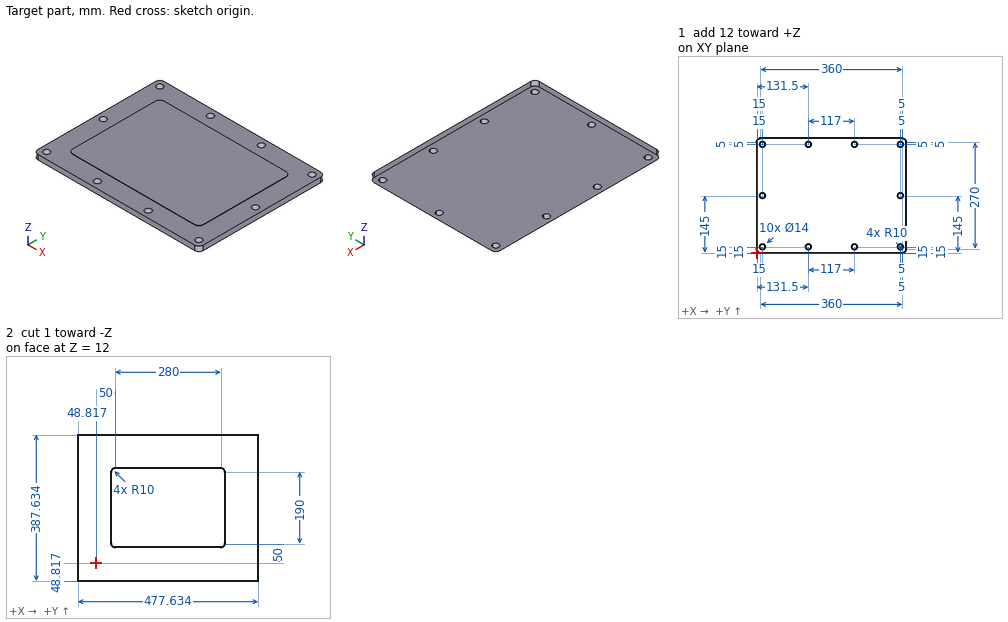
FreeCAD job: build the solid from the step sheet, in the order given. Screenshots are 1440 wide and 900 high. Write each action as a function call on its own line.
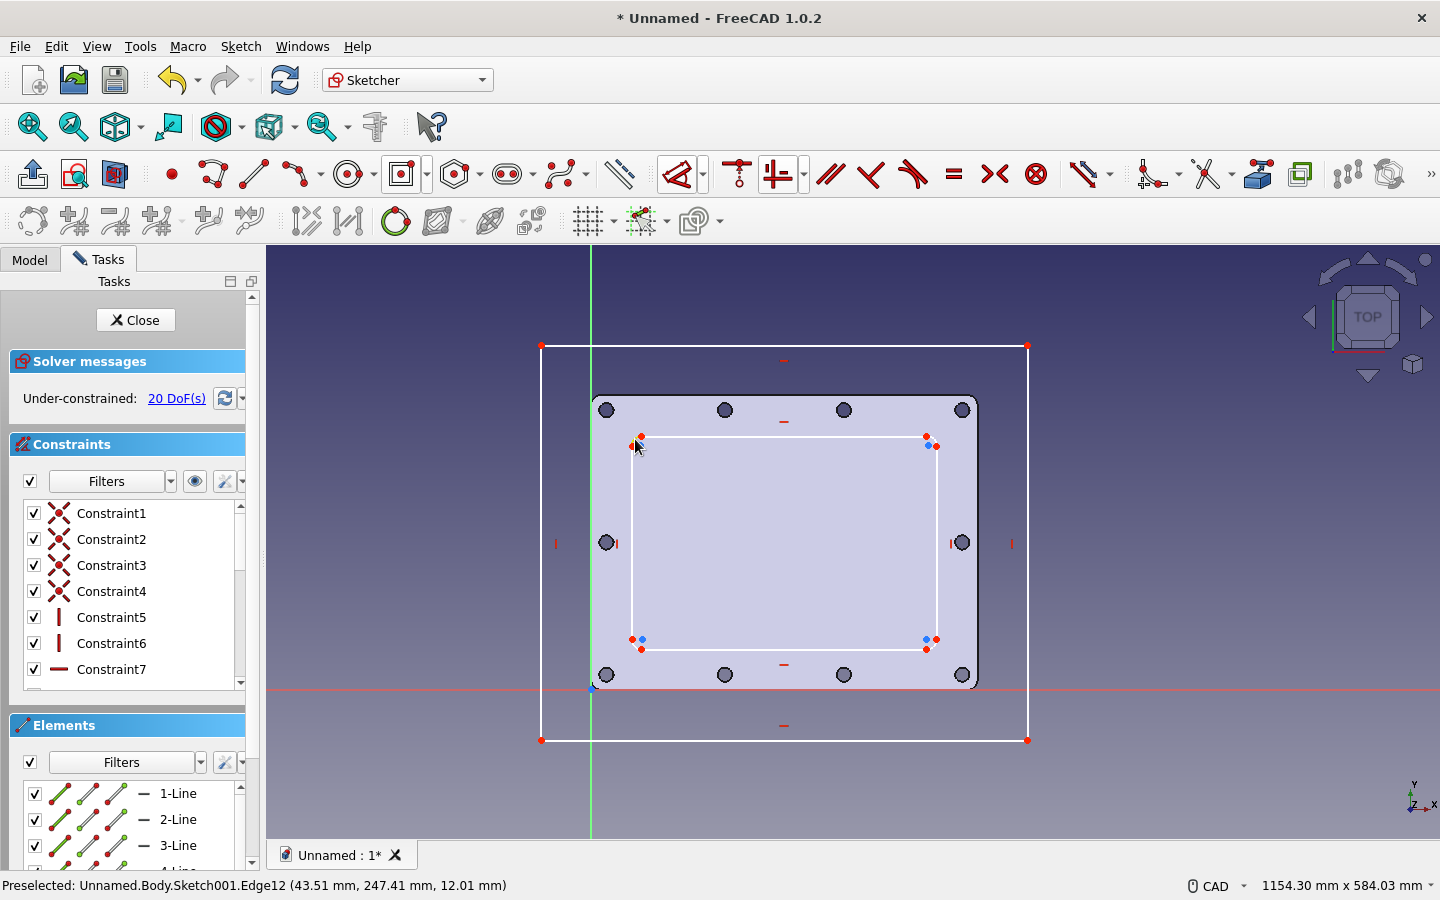
click(727, 437)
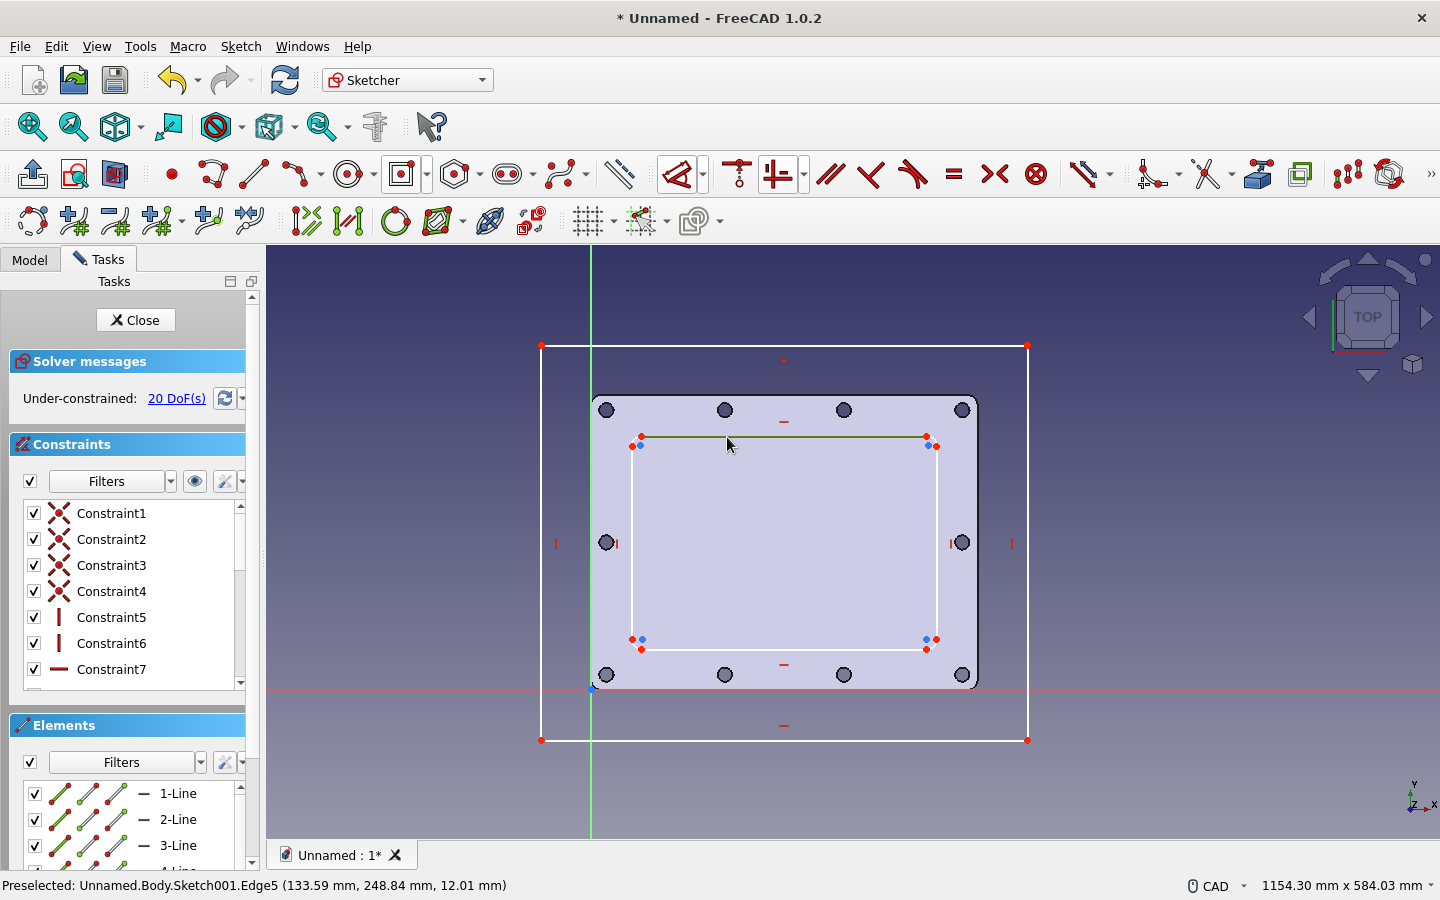
scroll(934, 439, up, 3)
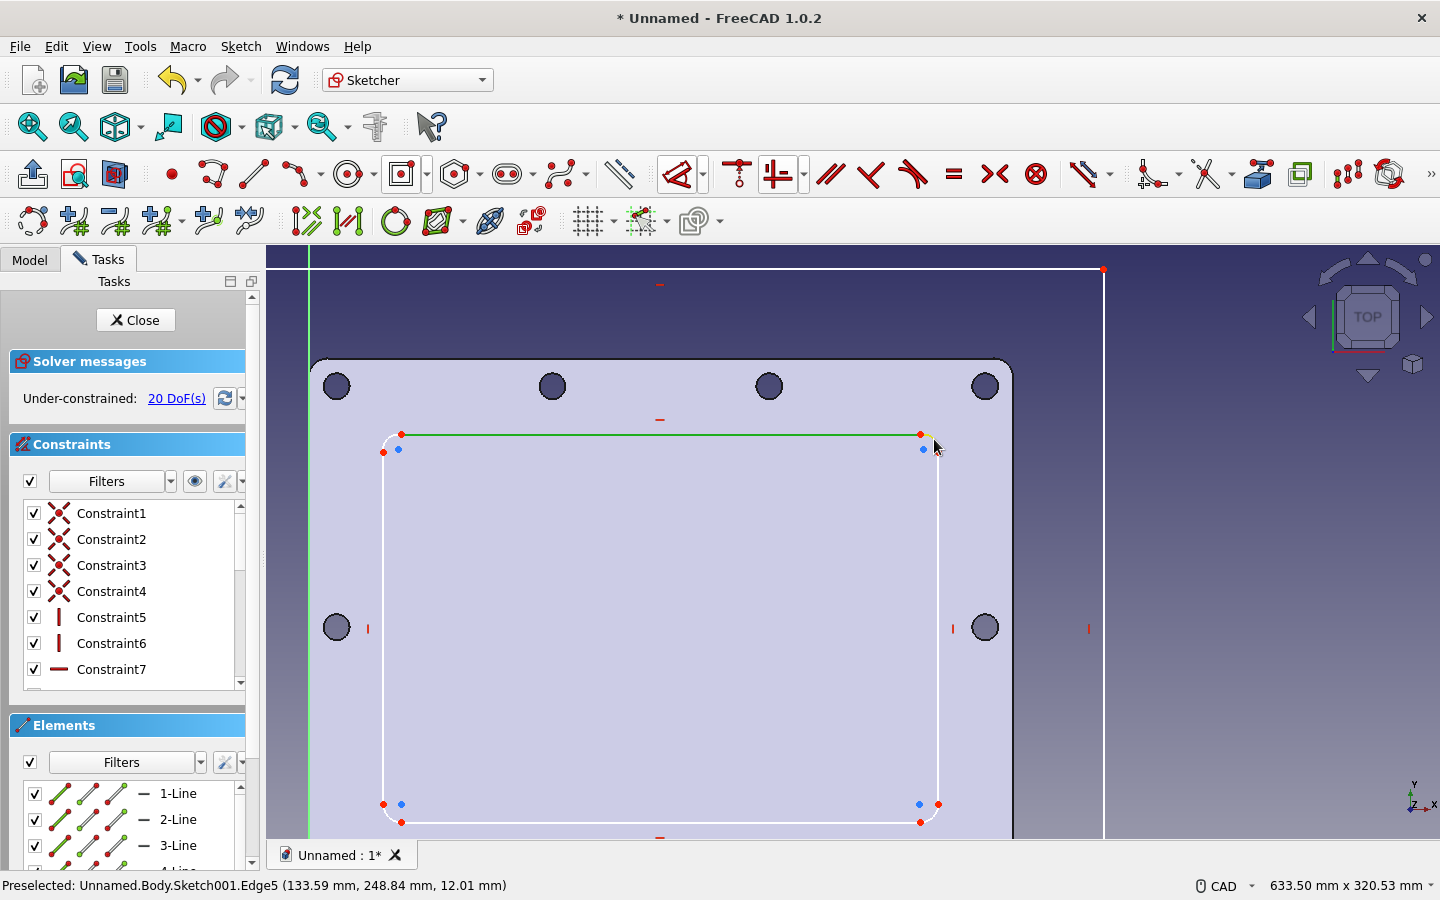
click(934, 439)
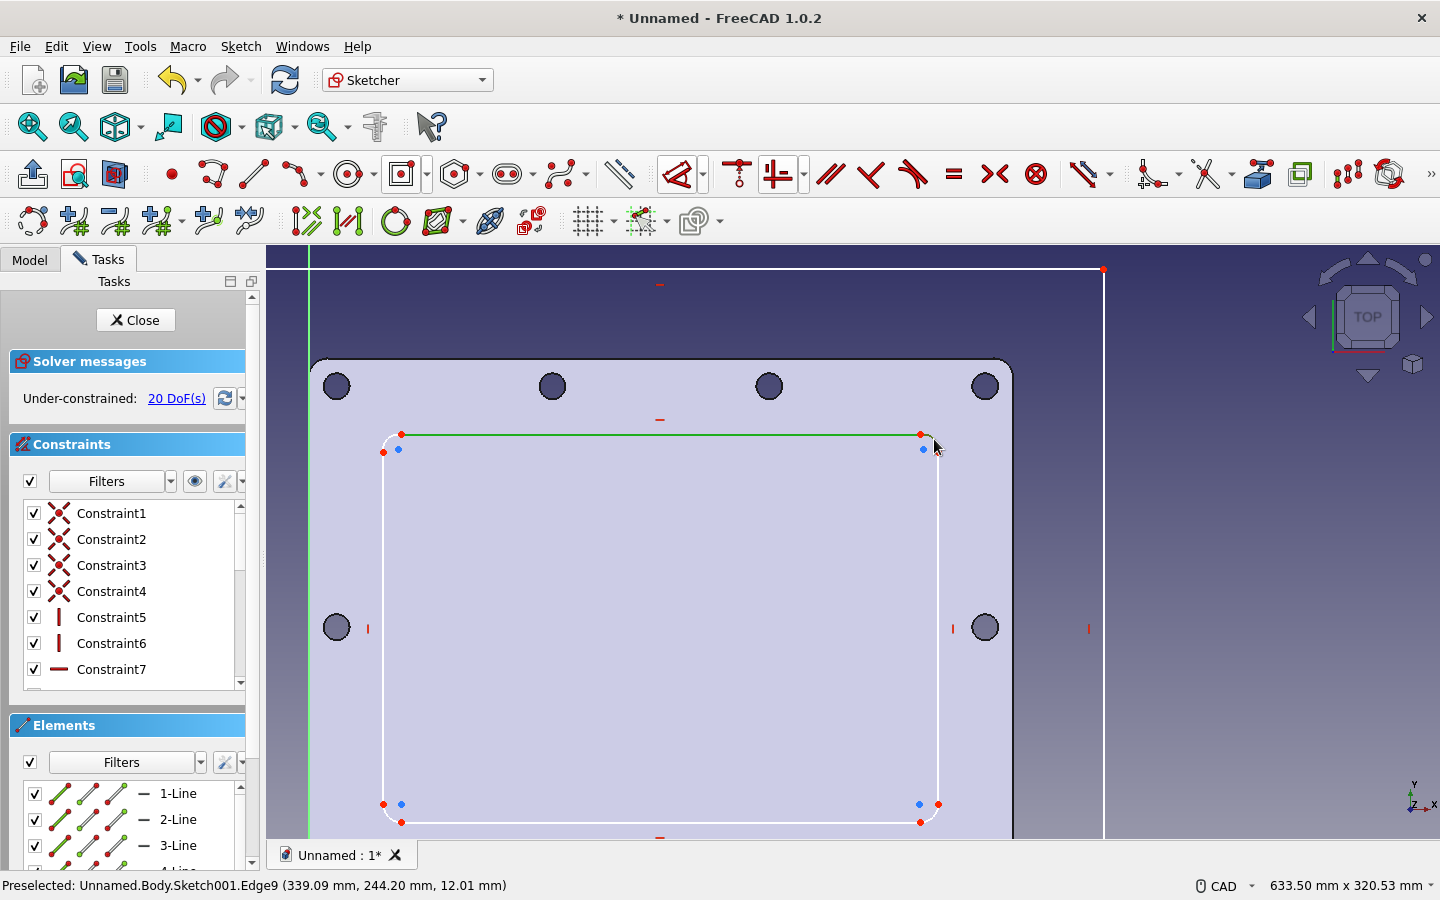
click(913, 174)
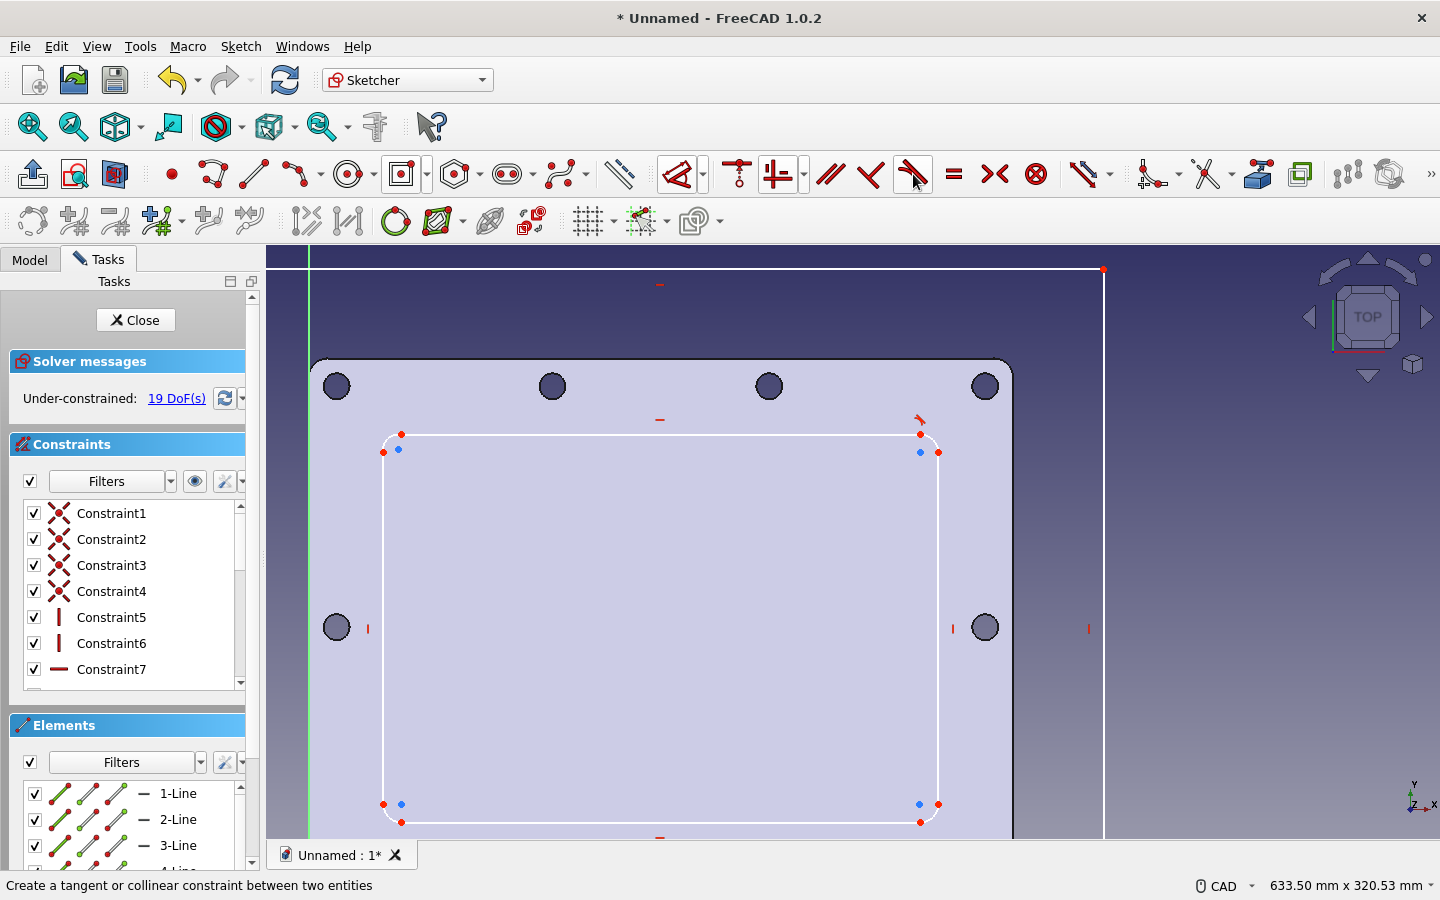
click(557, 435)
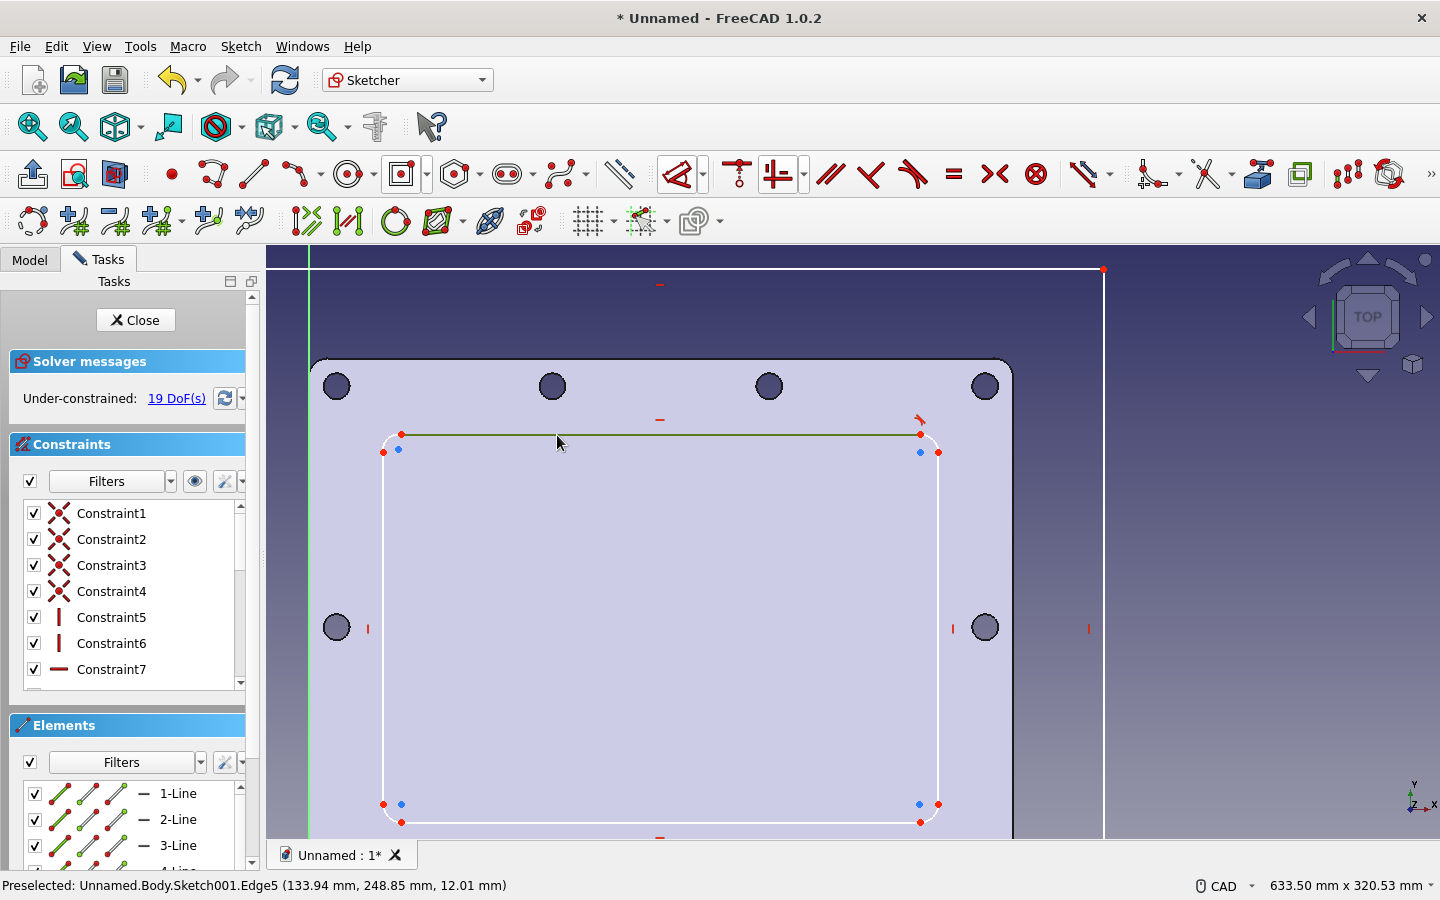
click(388, 439)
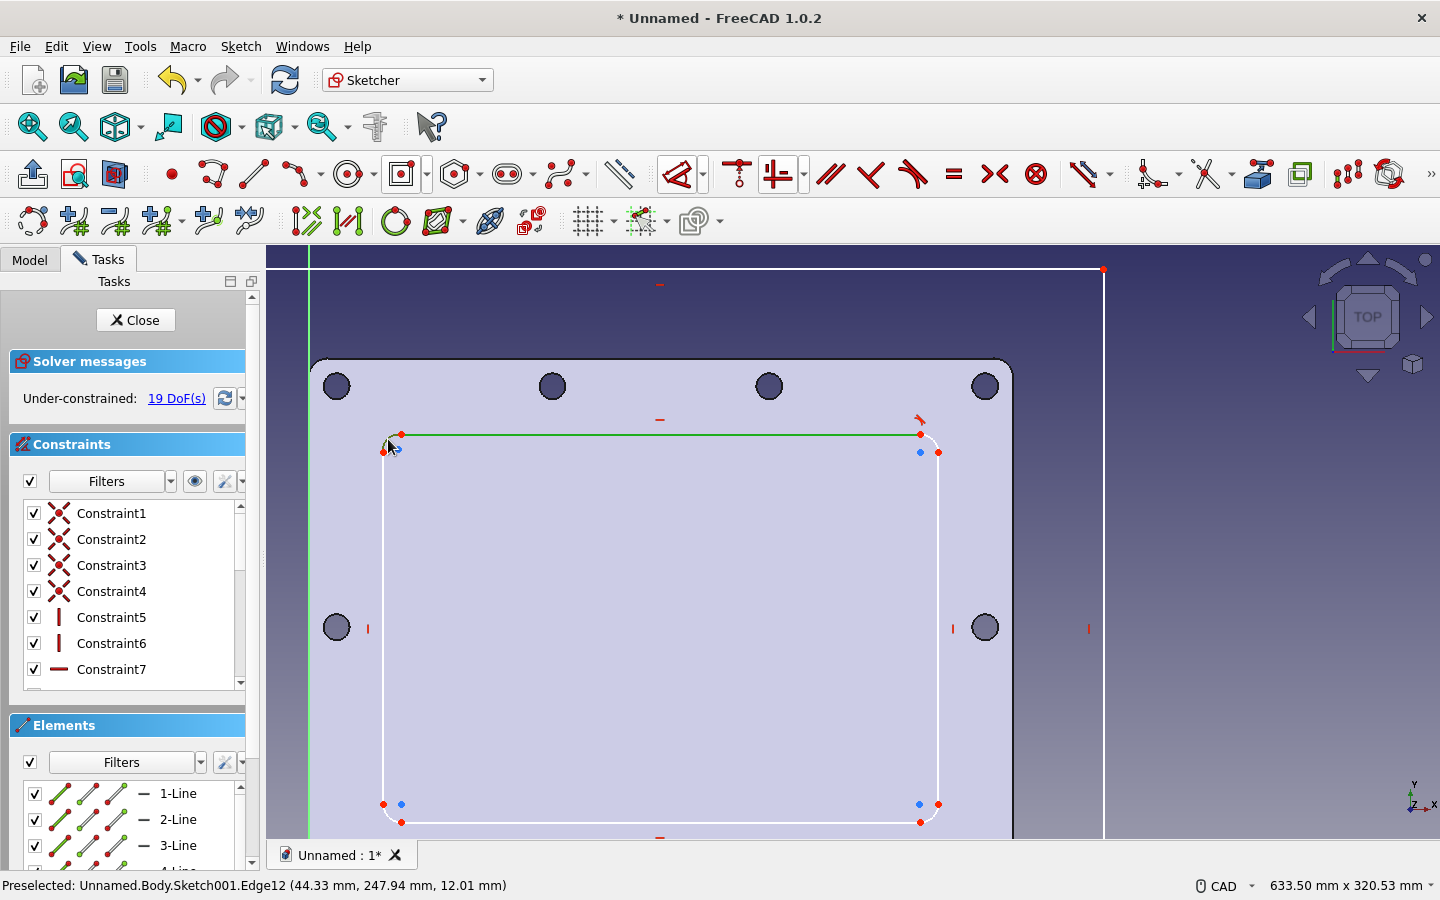
click(913, 174)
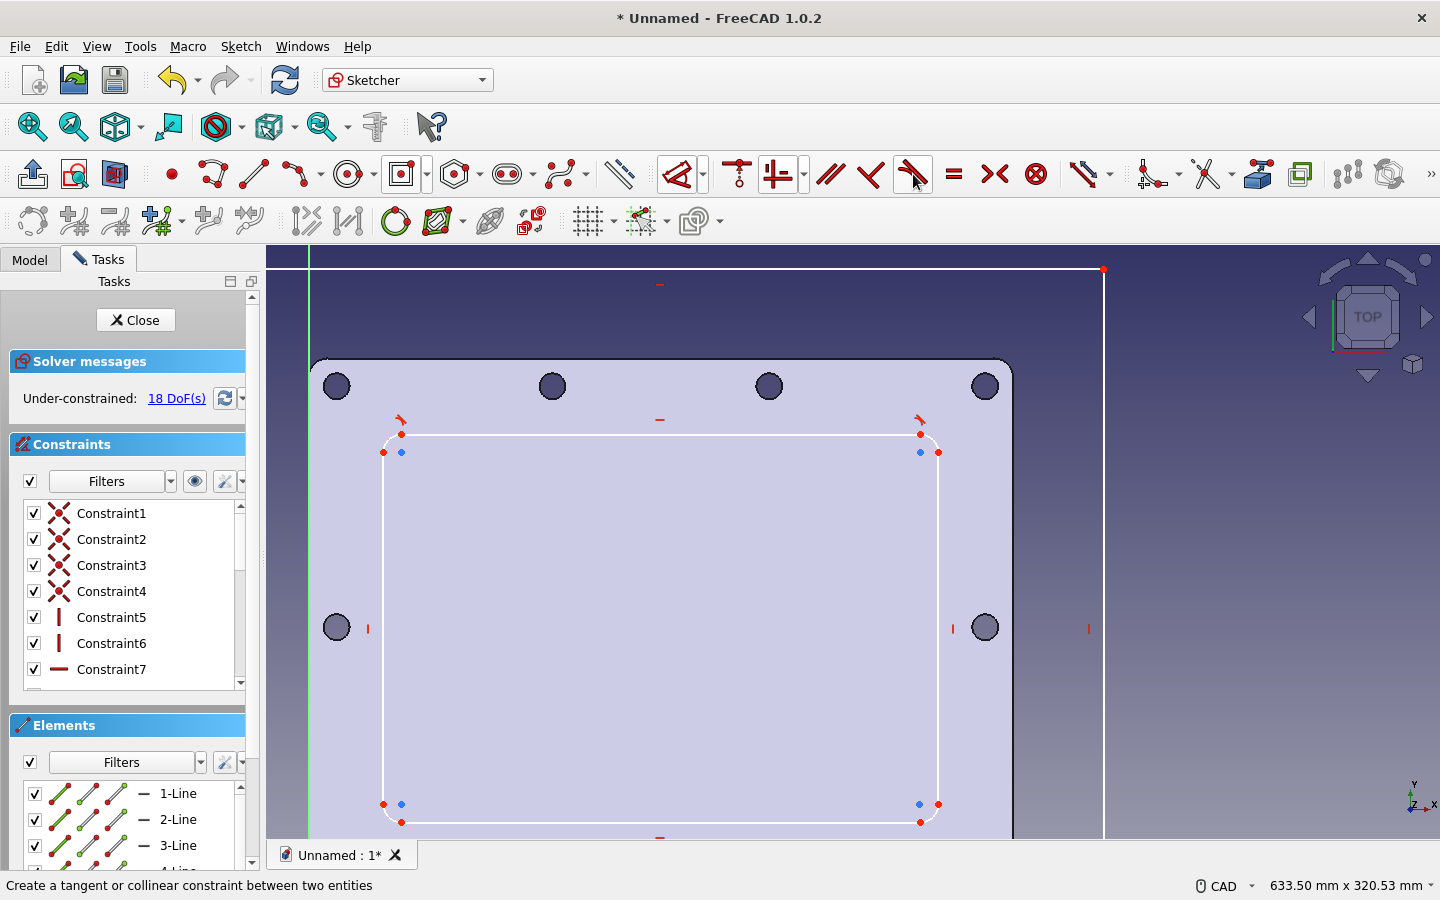
click(938, 558)